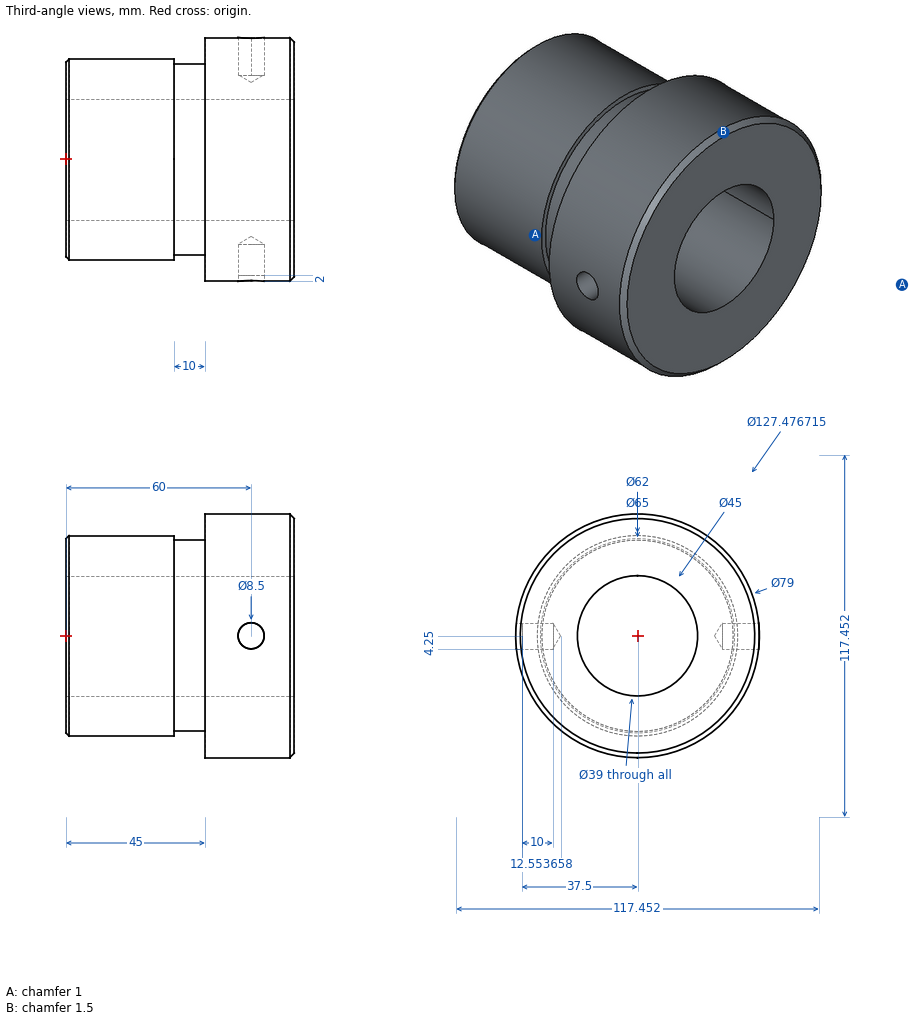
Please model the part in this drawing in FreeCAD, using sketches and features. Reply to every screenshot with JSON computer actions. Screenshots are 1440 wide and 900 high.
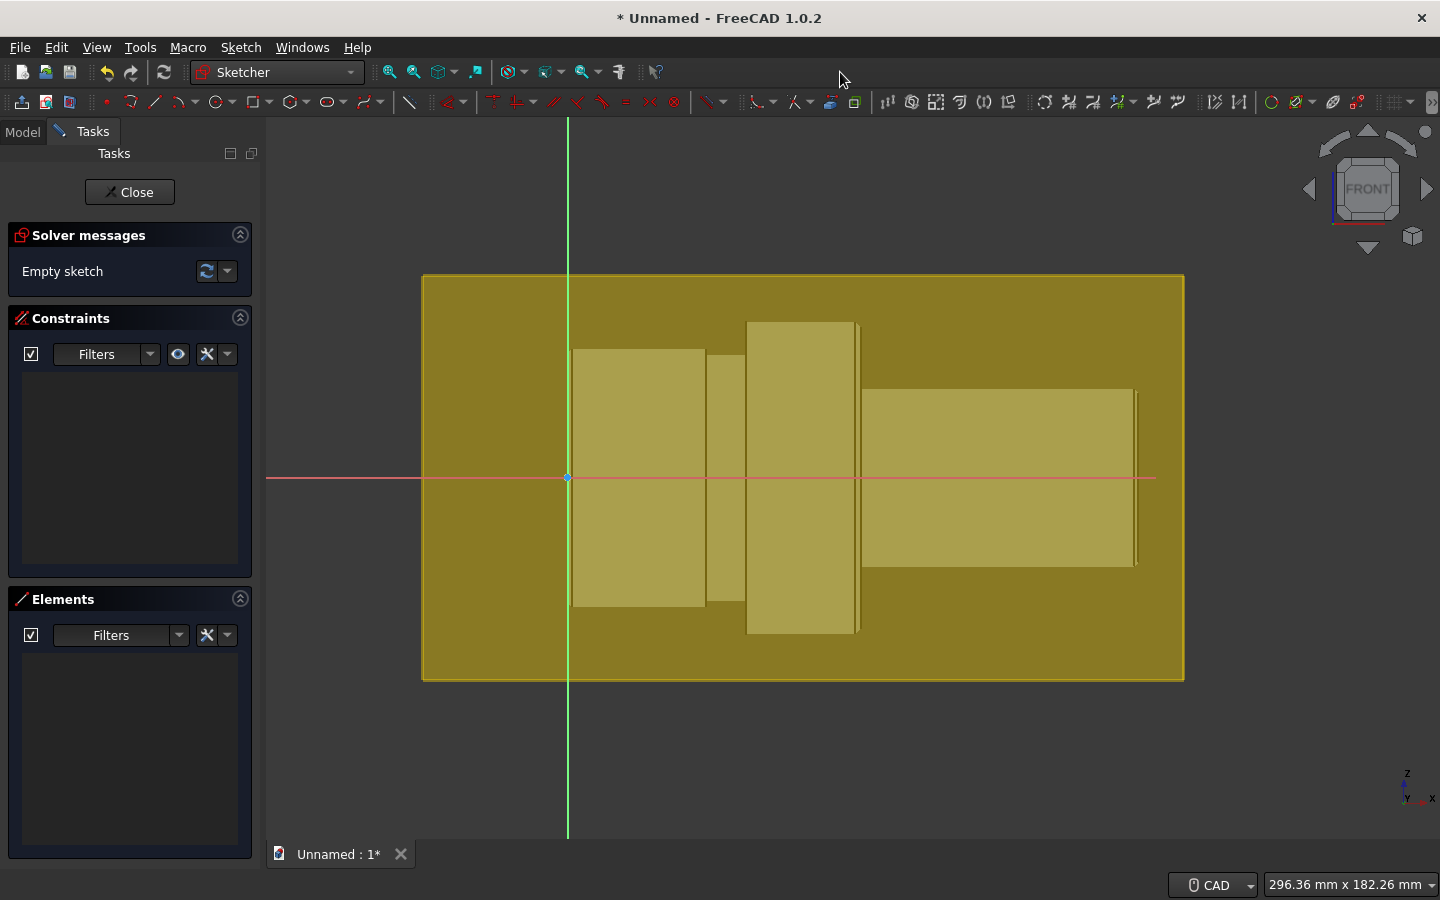
{"action": "scroll", "coordinate": [807, 478], "scroll_direction": "up", "scroll_amount": 13}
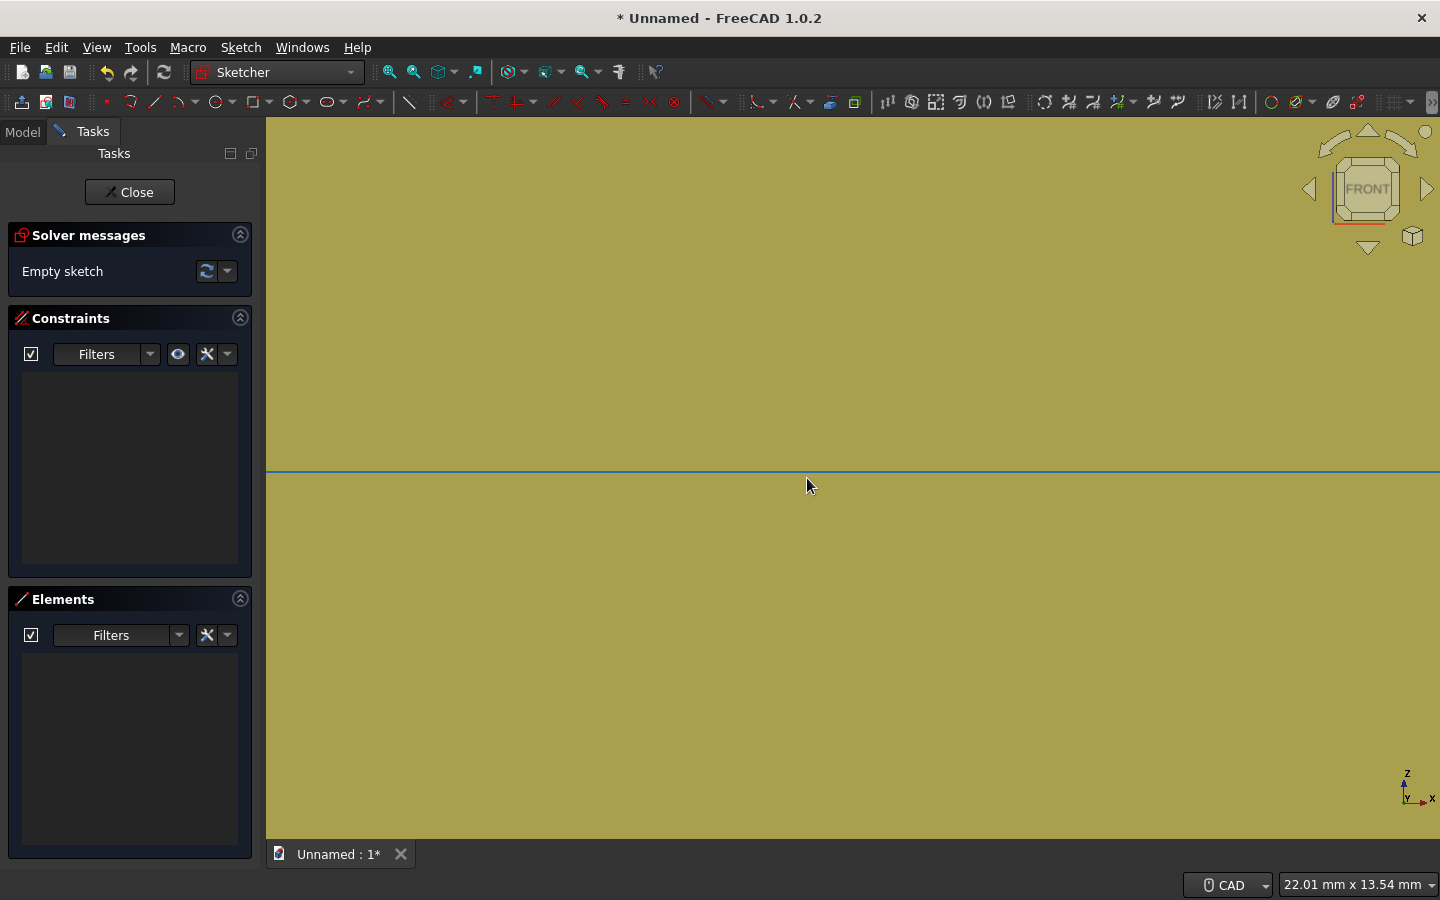
{"action": "key", "text": "g c"}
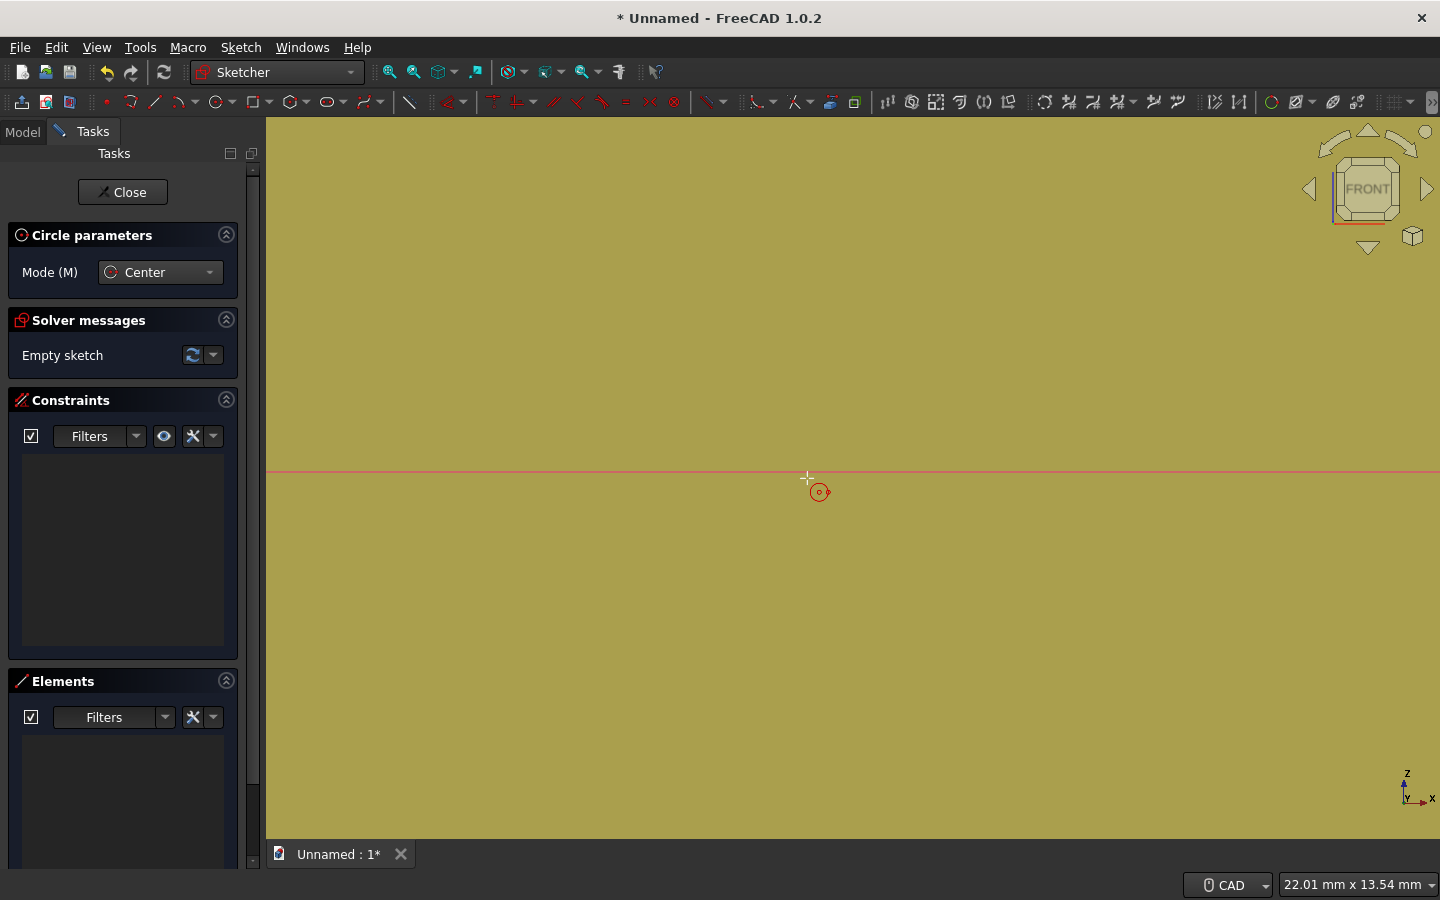
{"action": "left_click", "coordinate": [781, 472]}
{"action": "mouse_move", "coordinate": [941, 311]}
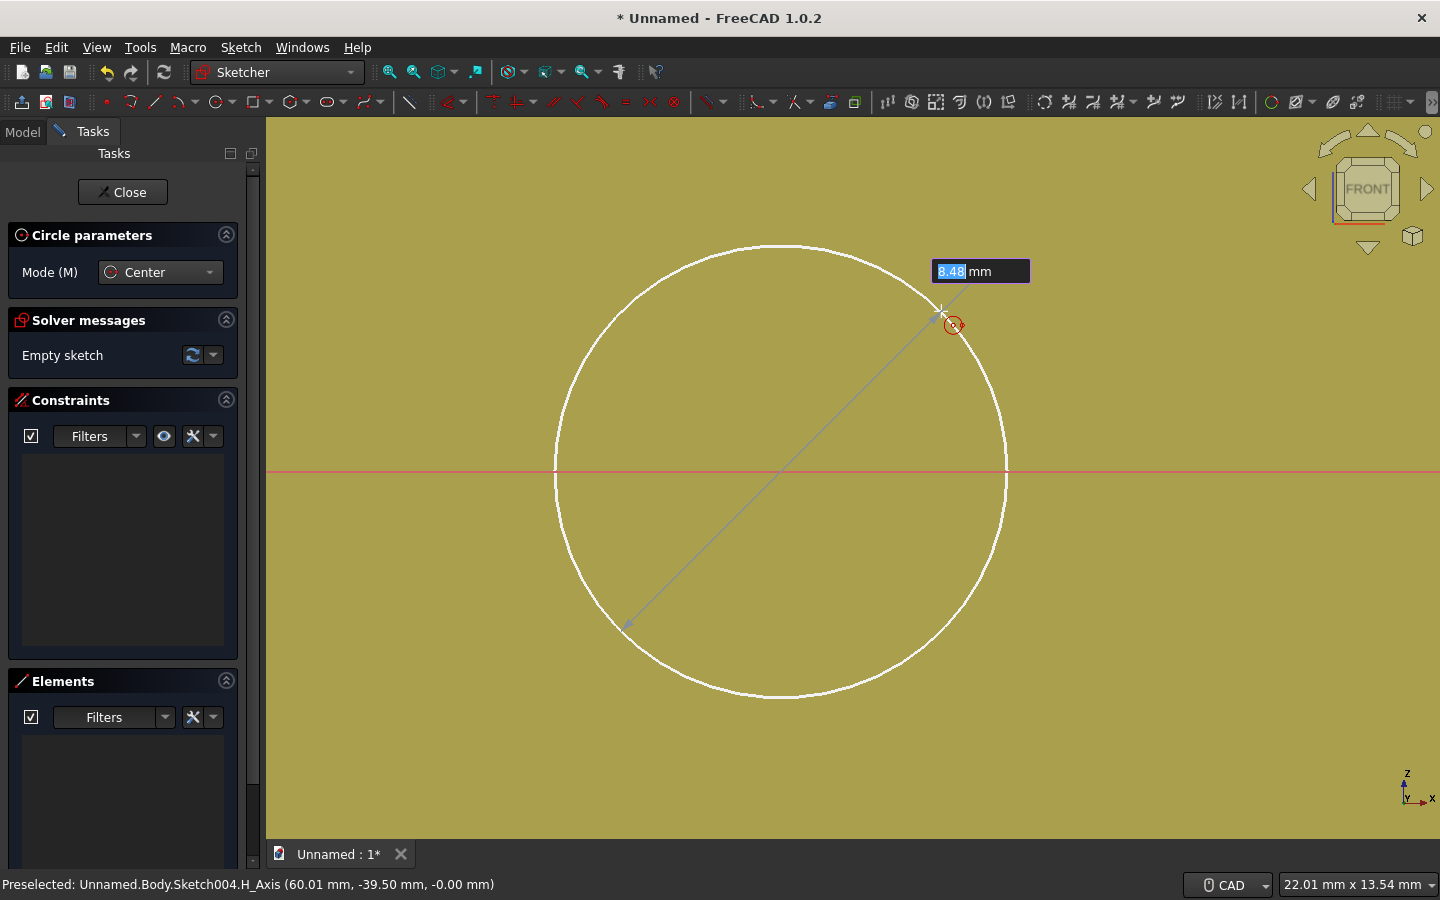
{"action": "type", "text": "8.5"}
{"action": "key", "text": "Return"}
{"action": "key", "text": "Escape"}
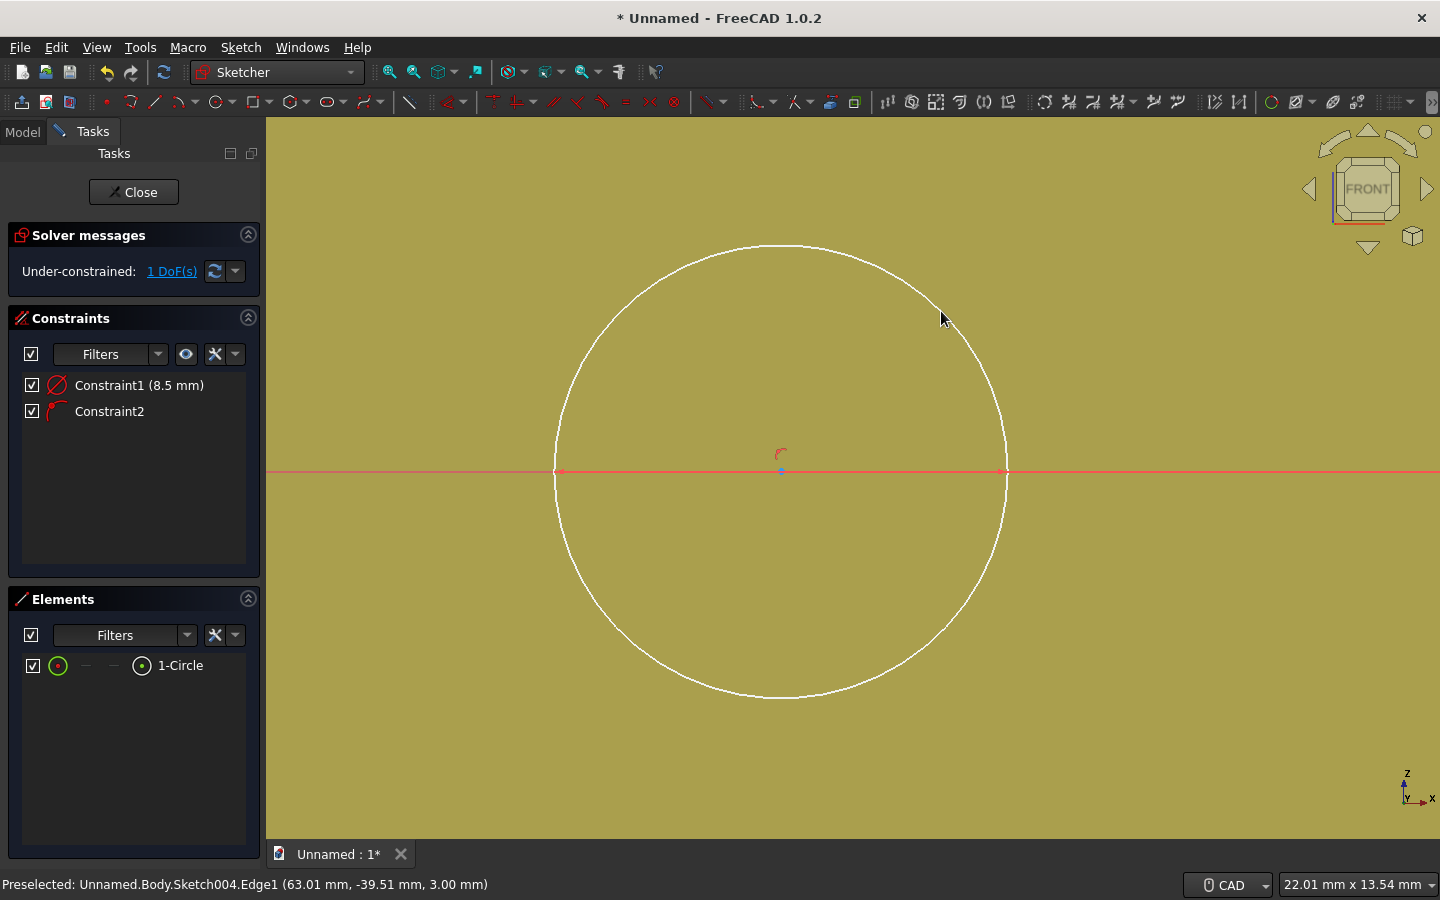
{"action": "key", "text": "d"}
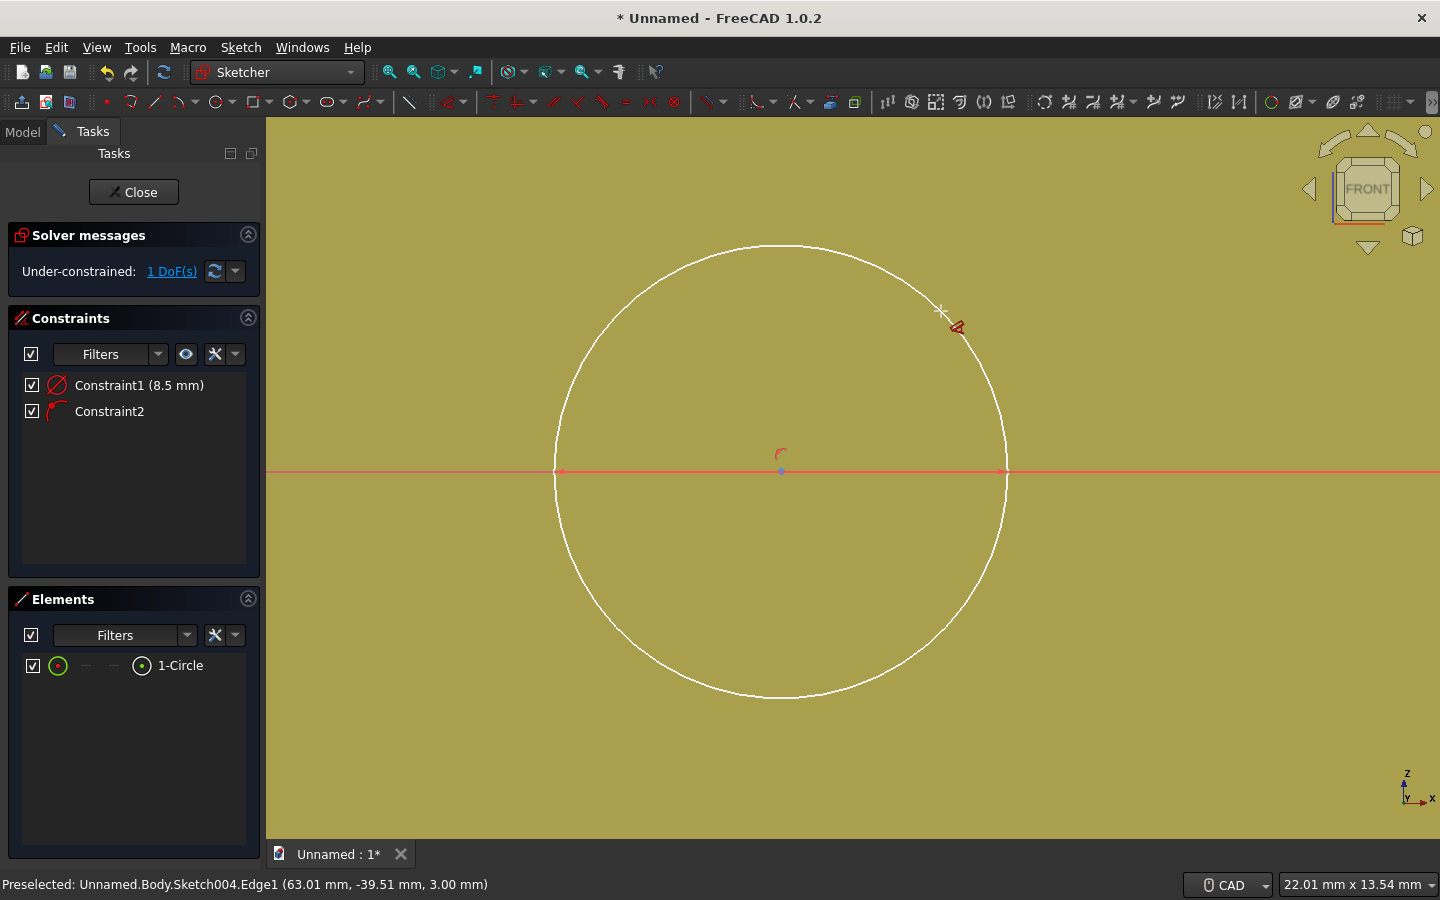
{"action": "left_click", "coordinate": [781, 472]}
{"action": "left_click", "coordinate": [538, 506]}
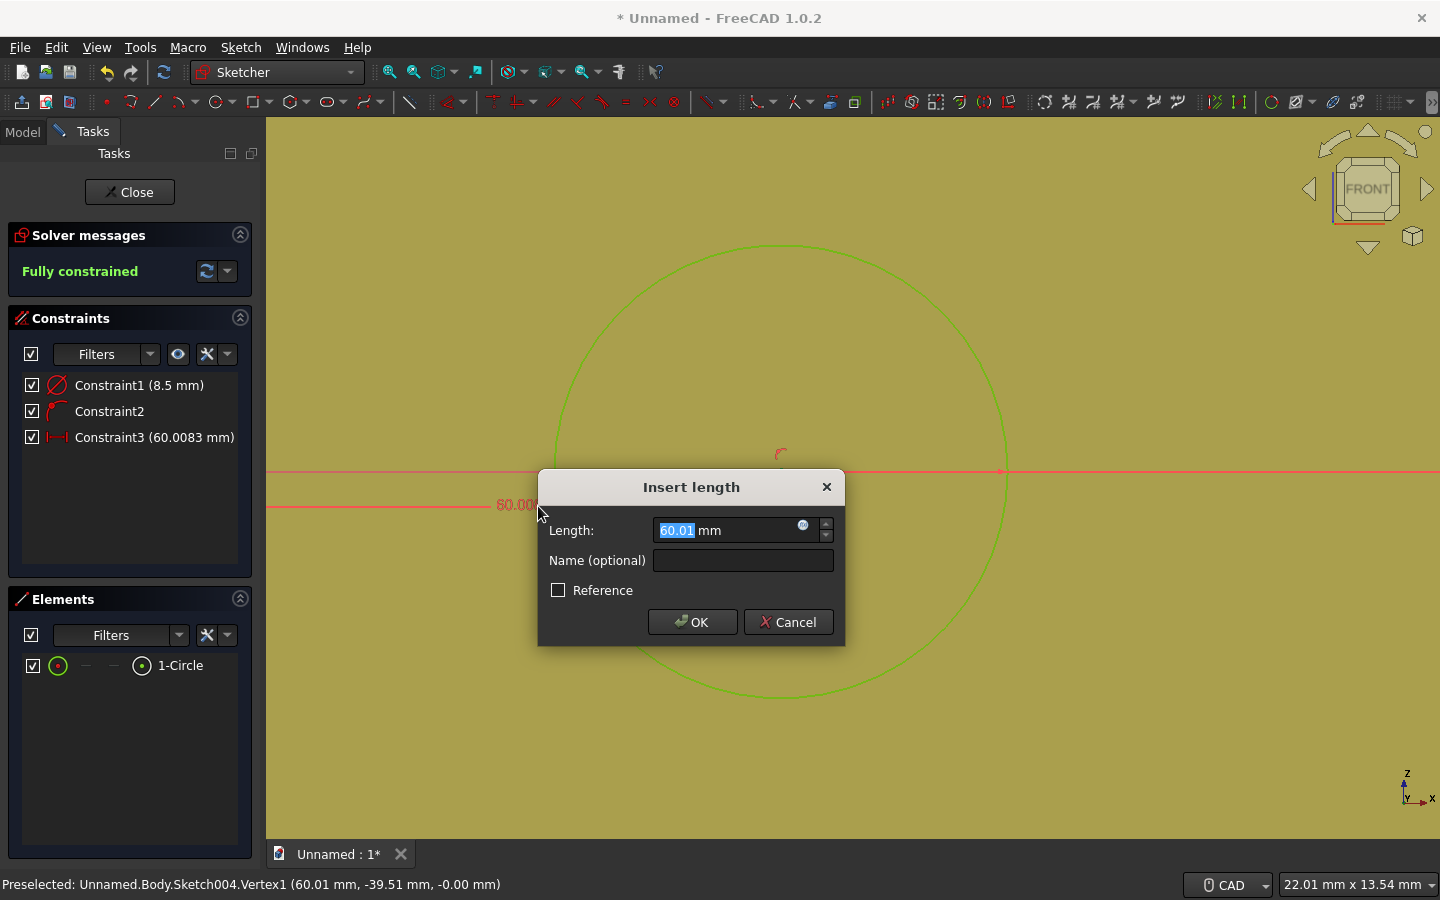
{"action": "type", "text": "60"}
{"action": "key", "text": "Return"}
{"action": "key", "text": "Escape"}